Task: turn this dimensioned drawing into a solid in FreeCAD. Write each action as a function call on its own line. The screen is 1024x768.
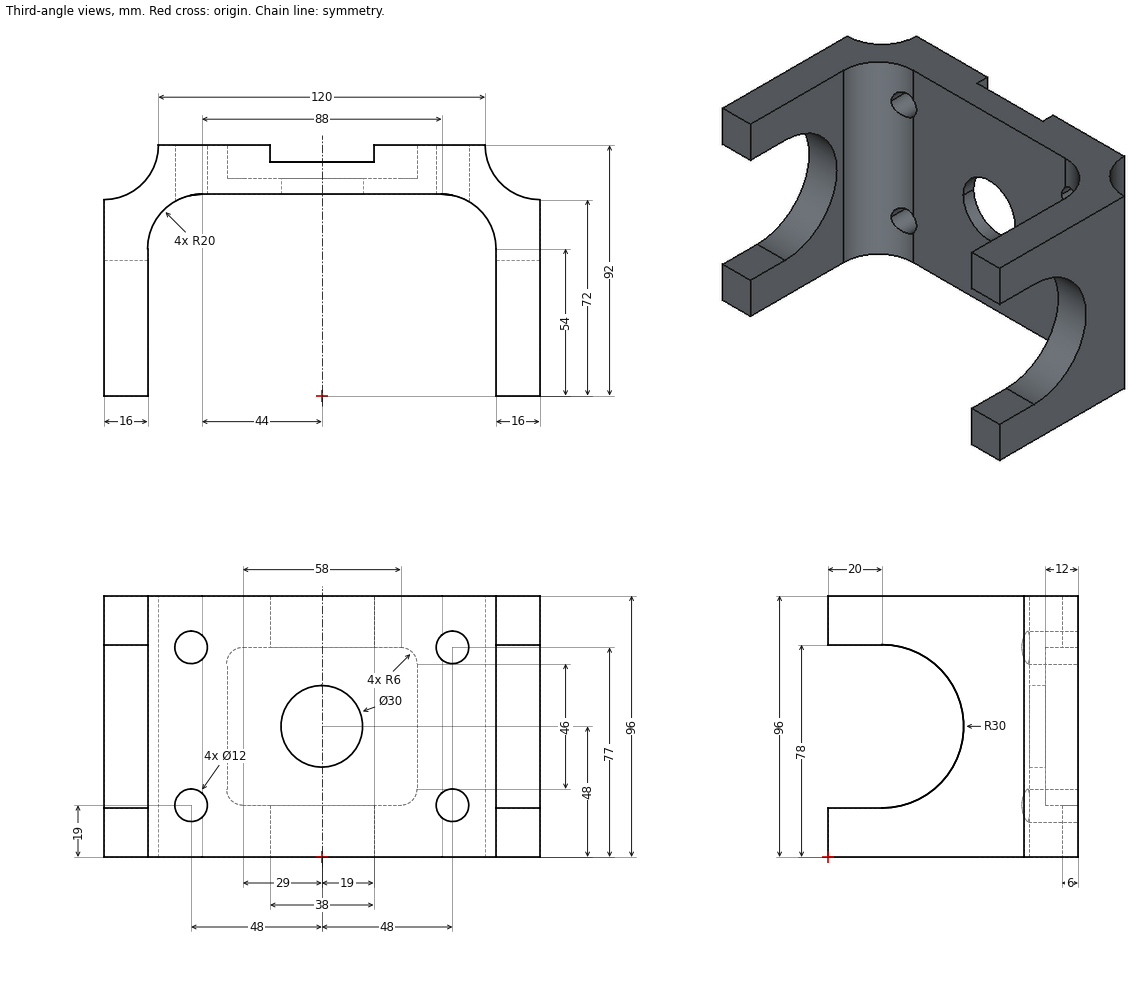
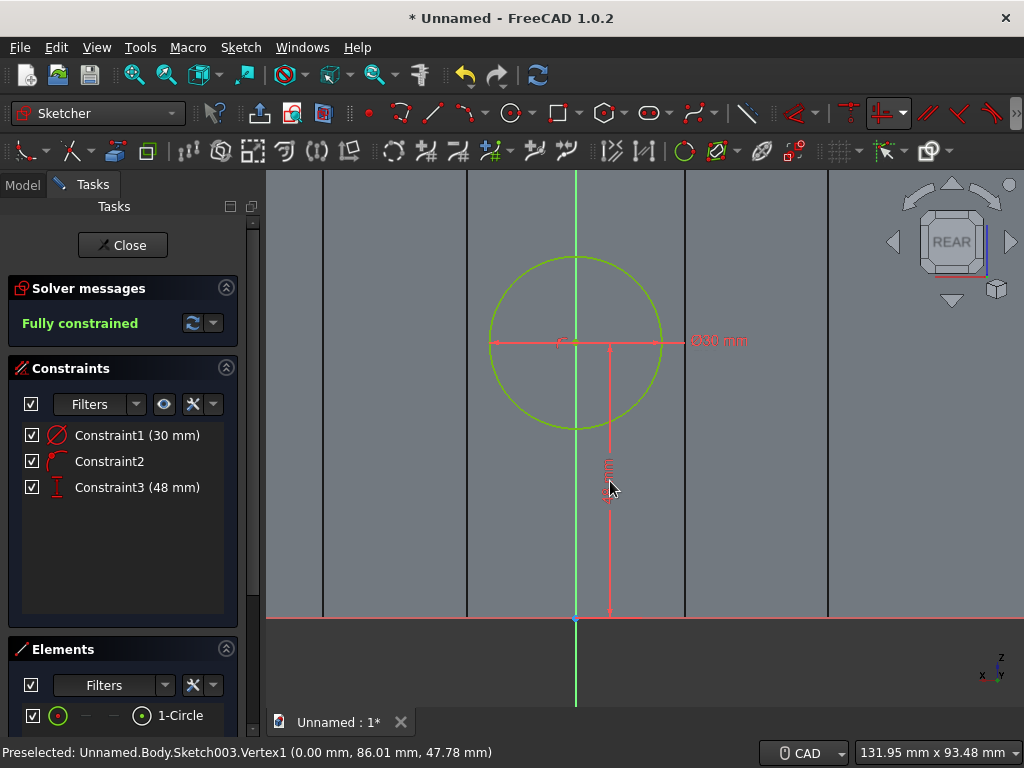
click(123, 245)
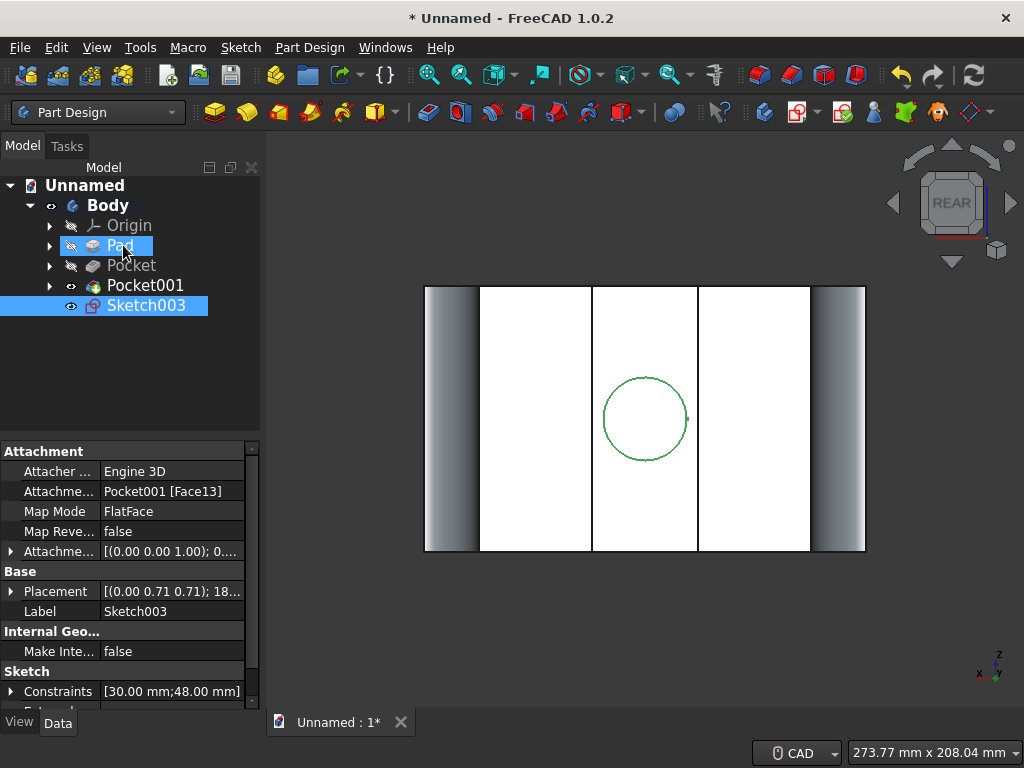
click(430, 112)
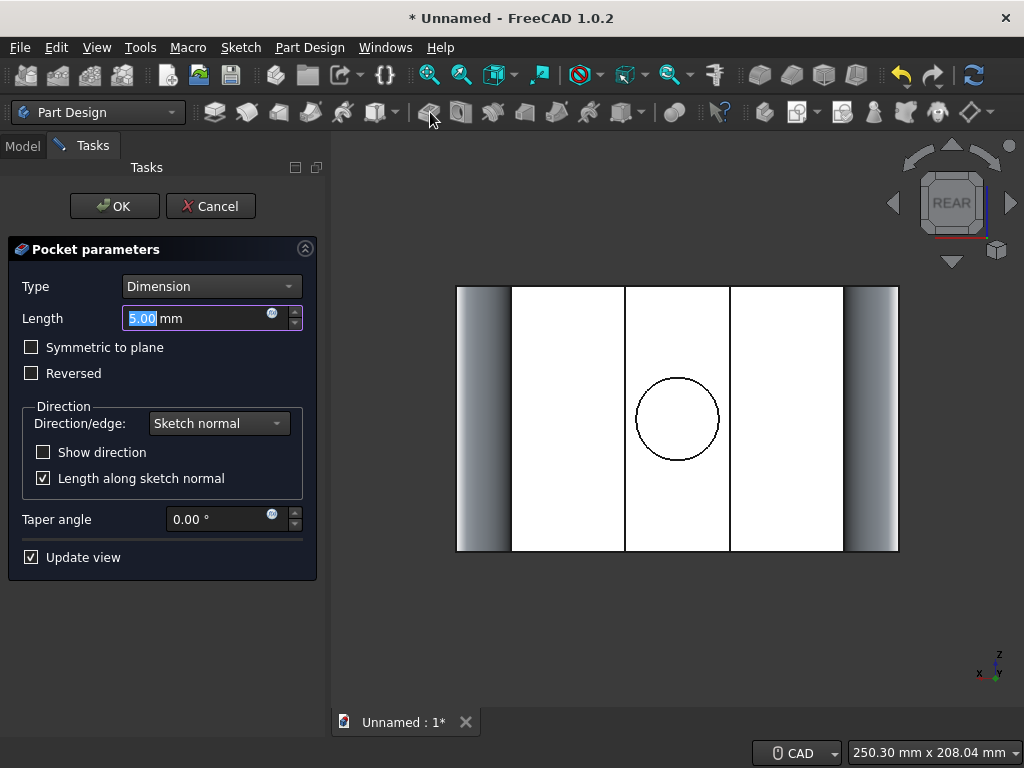
click(212, 286)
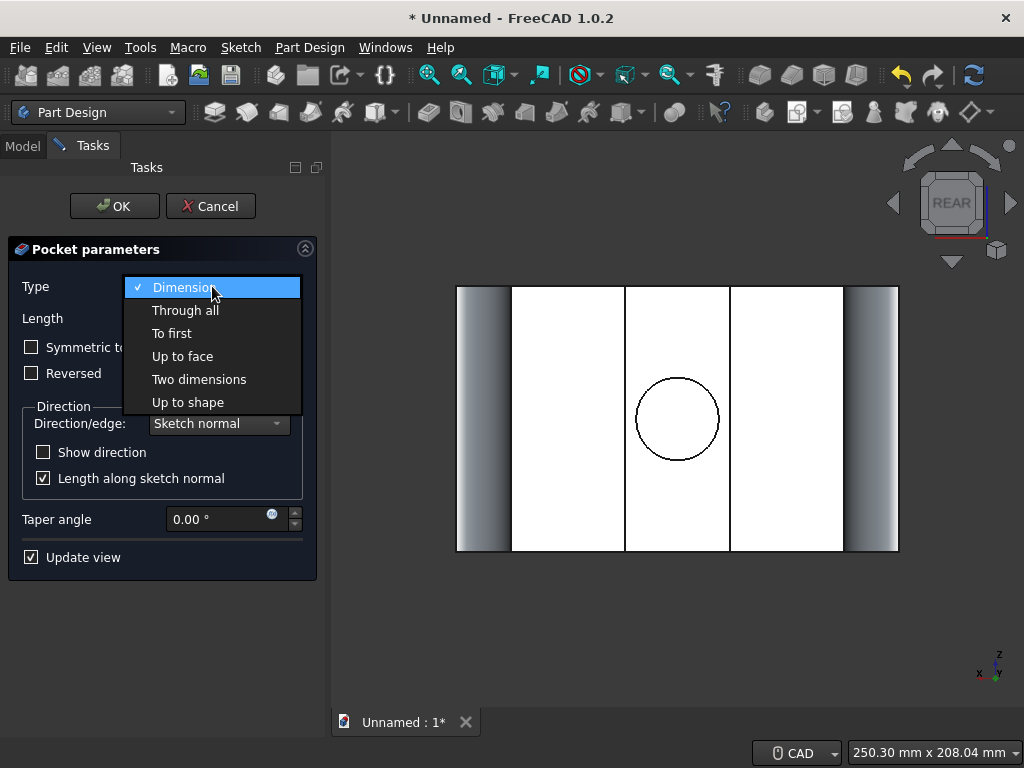
click(212, 310)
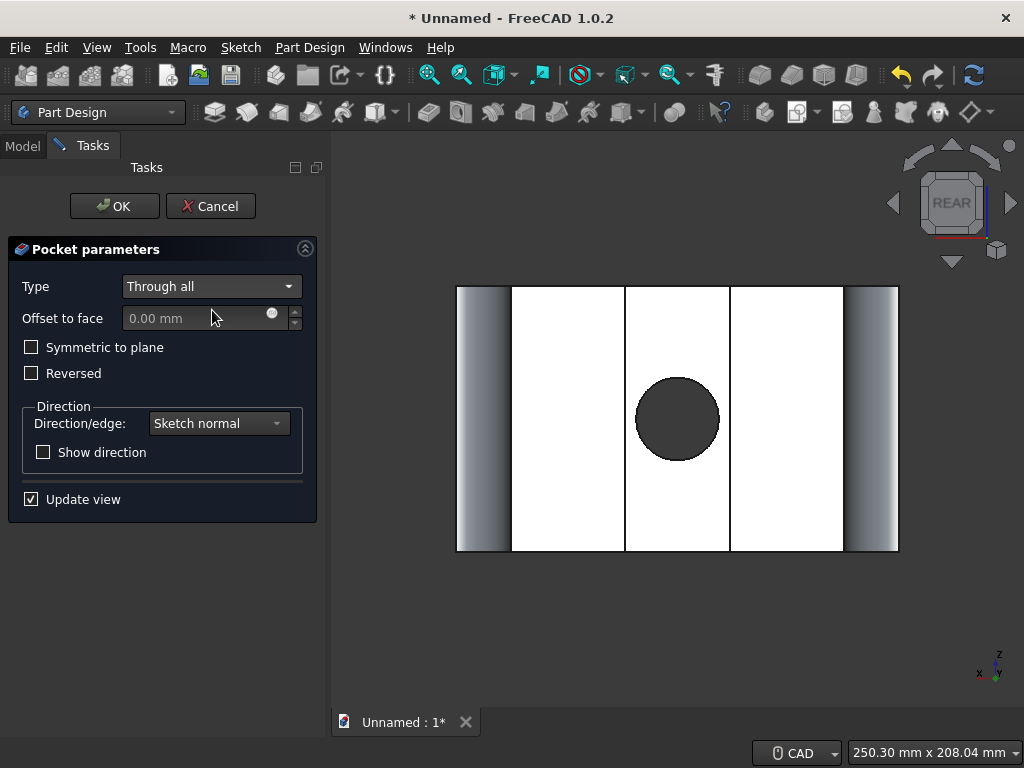
click(115, 206)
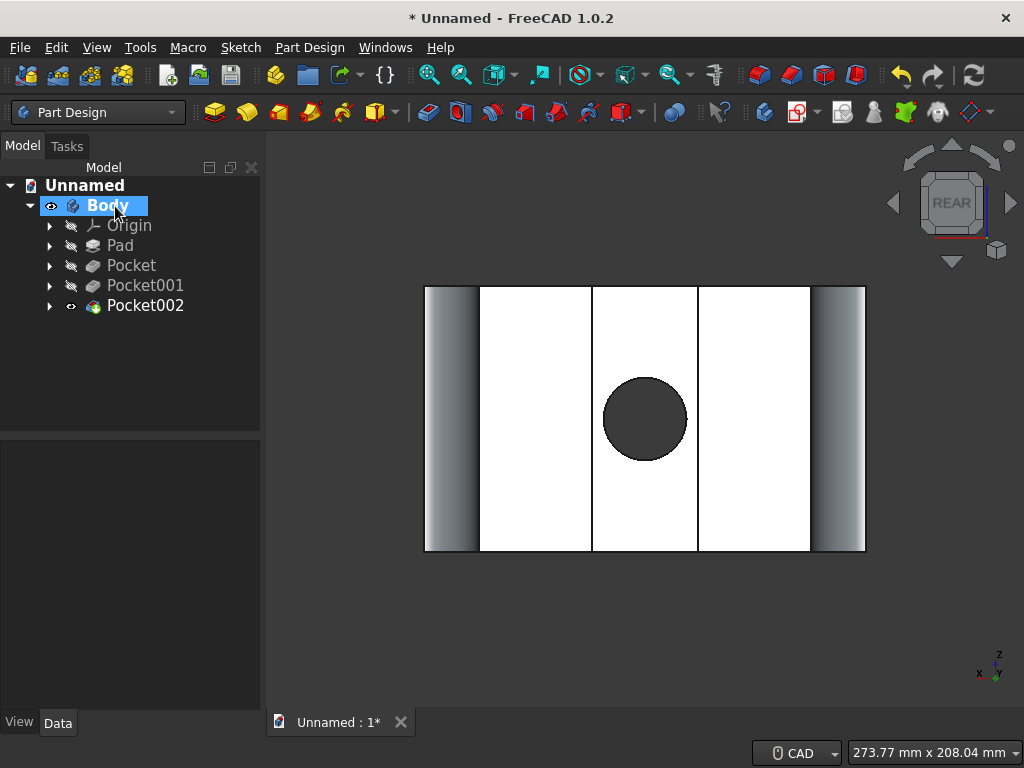
click(536, 342)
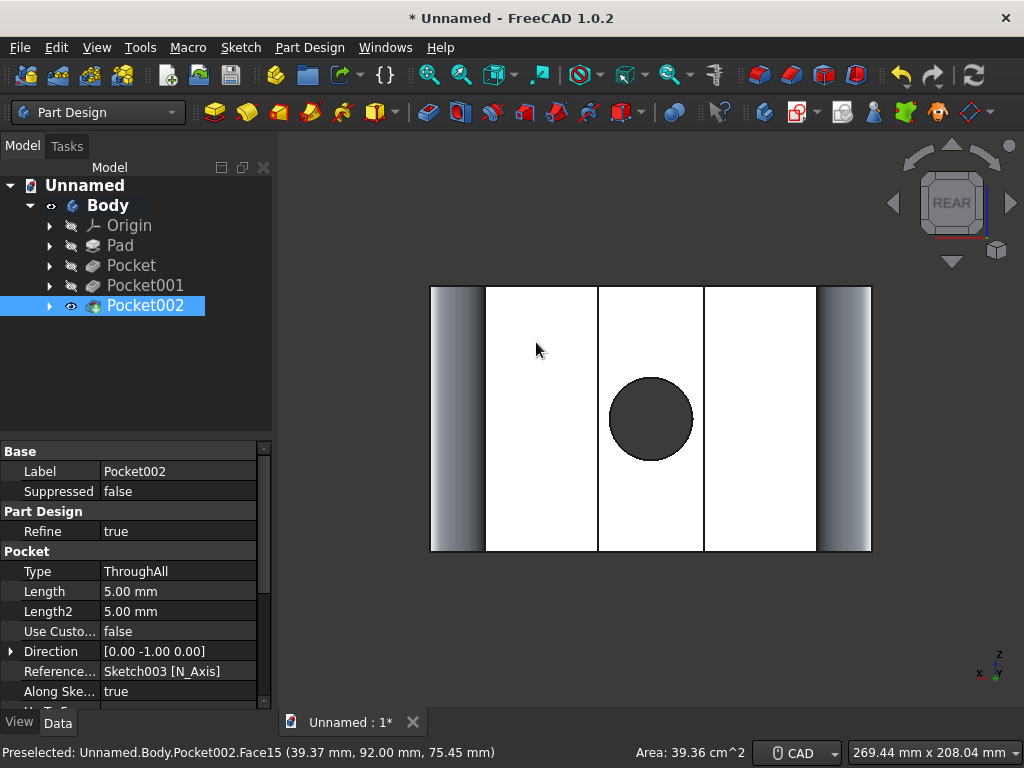
click(798, 112)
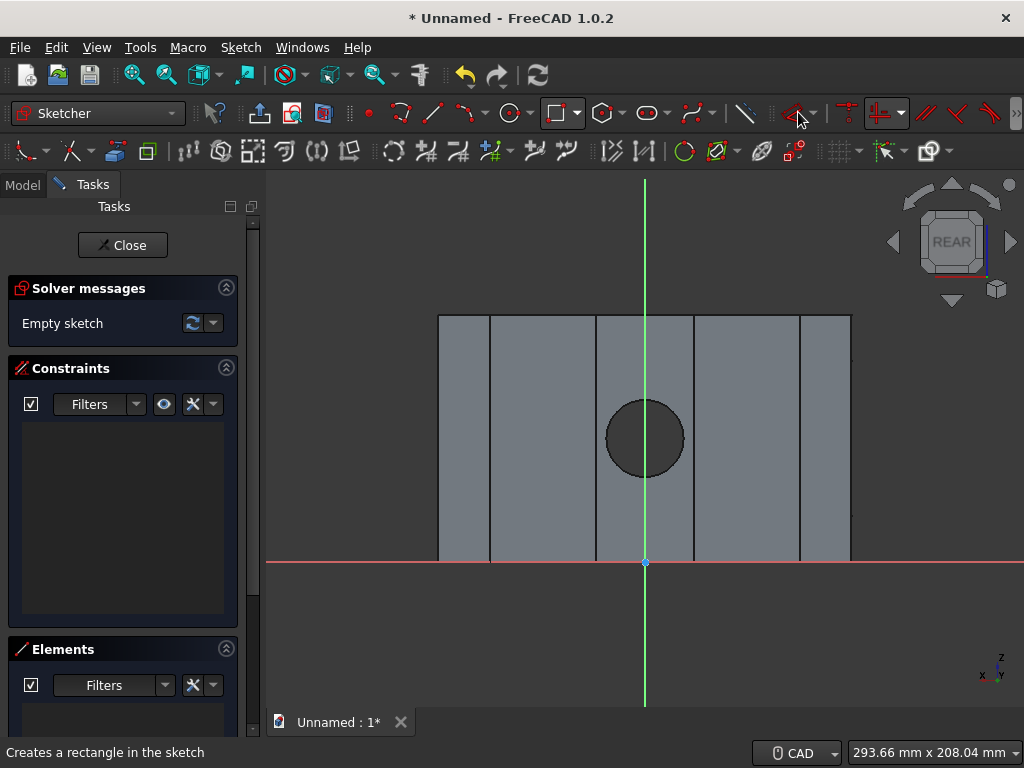
scroll(784, 489, up, 2)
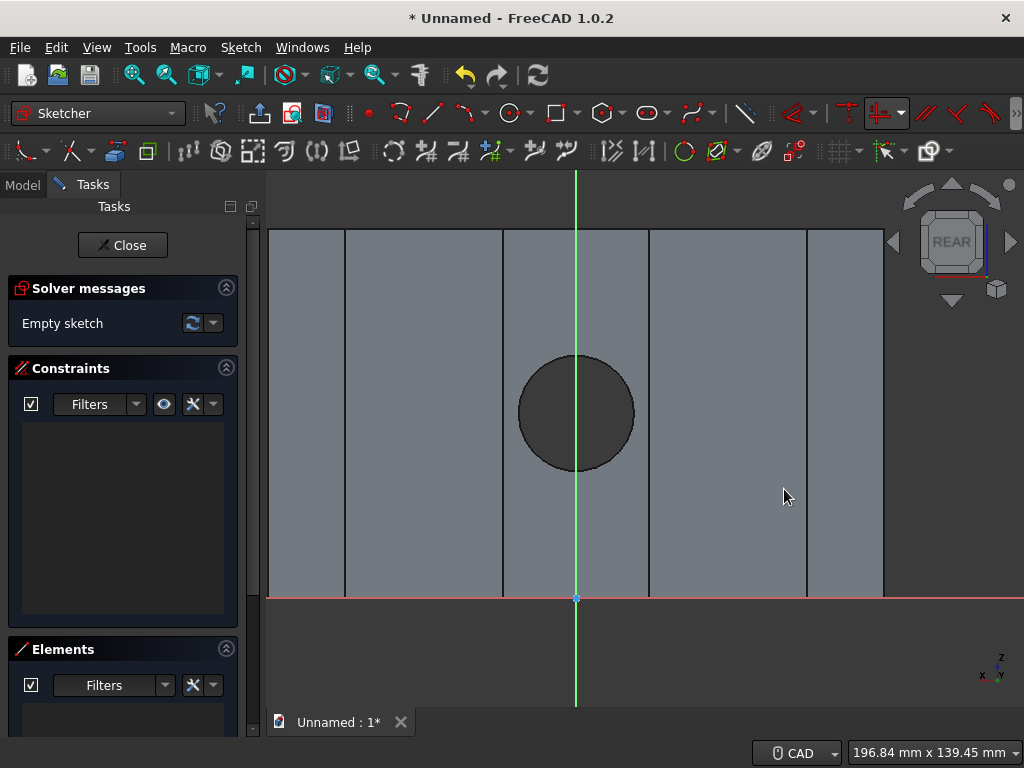
click(510, 114)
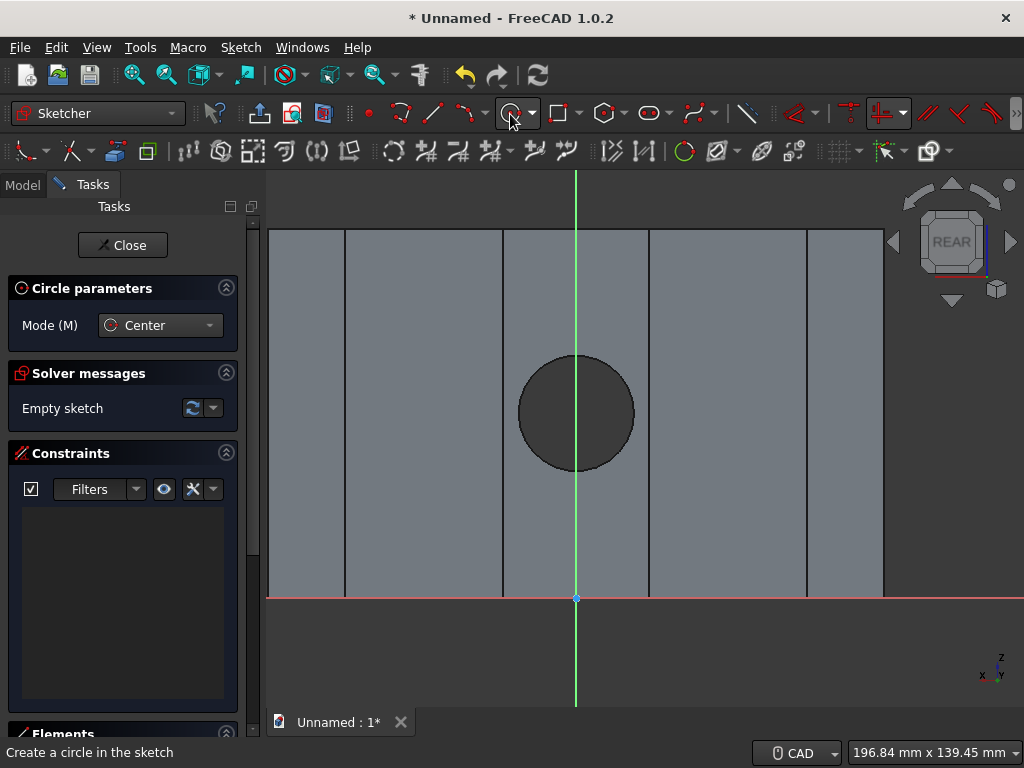
click(761, 525)
move(777, 509)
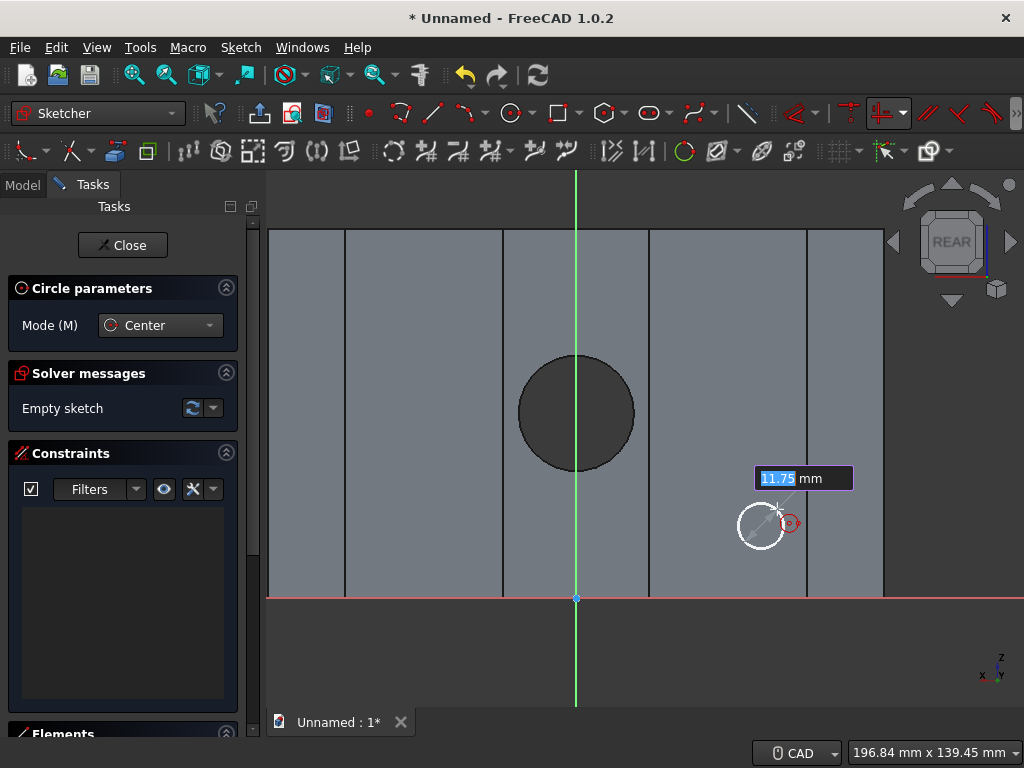
text(12)
key(Return)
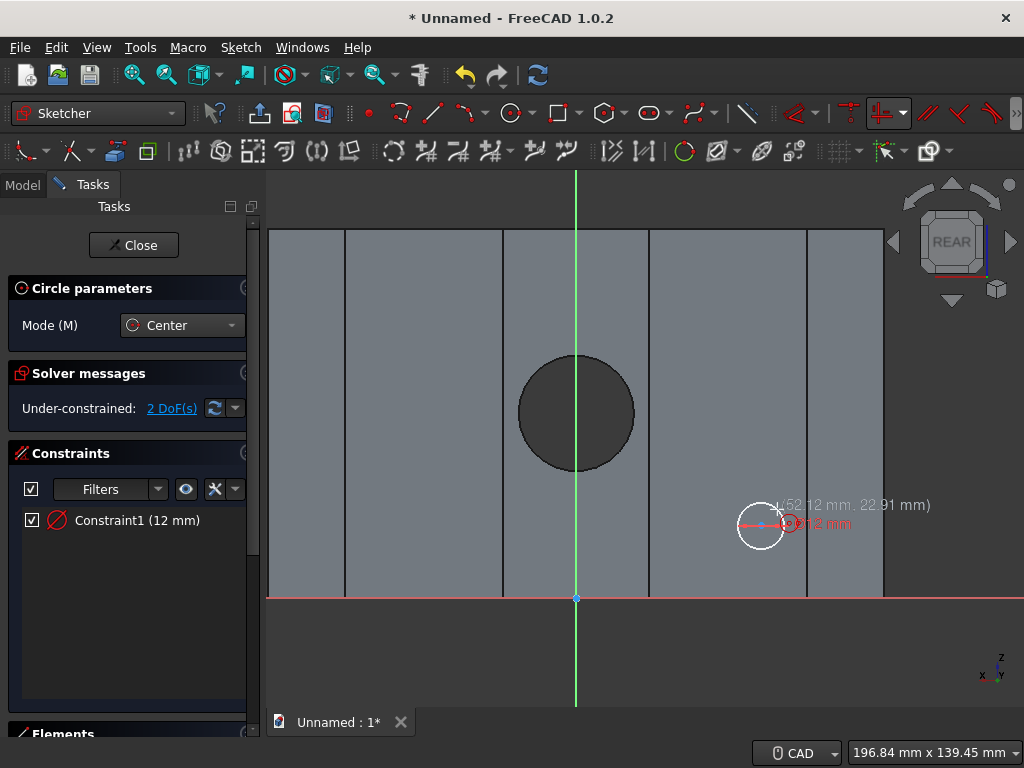
click(391, 525)
move(408, 509)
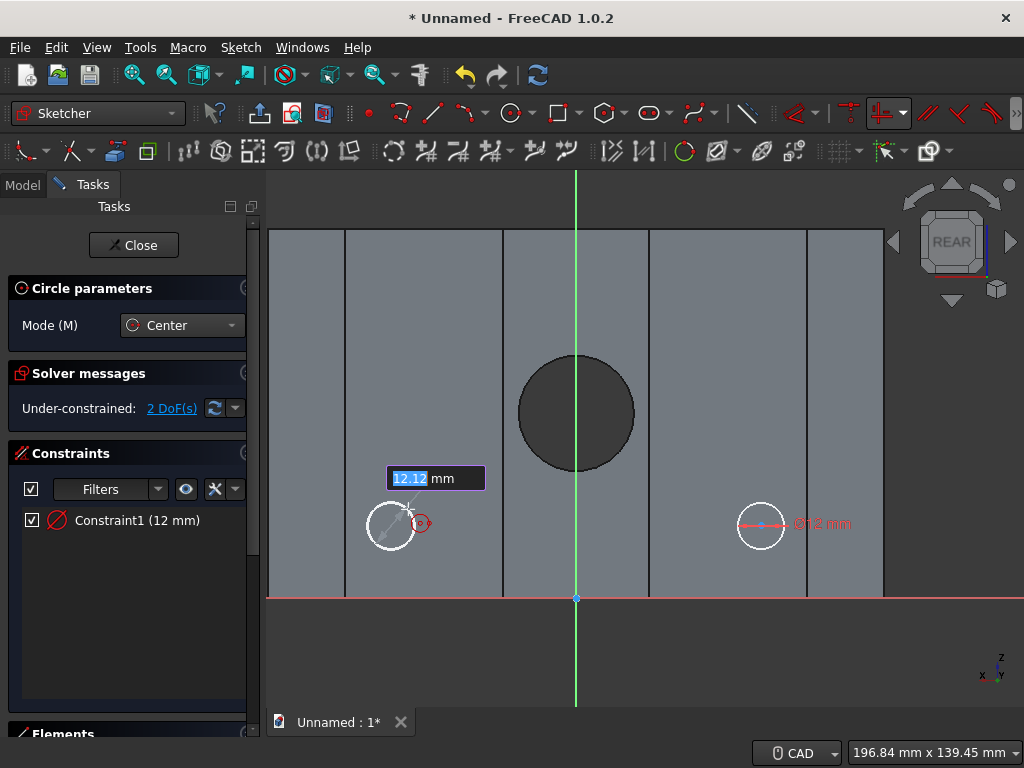
text(12)
key(Return)